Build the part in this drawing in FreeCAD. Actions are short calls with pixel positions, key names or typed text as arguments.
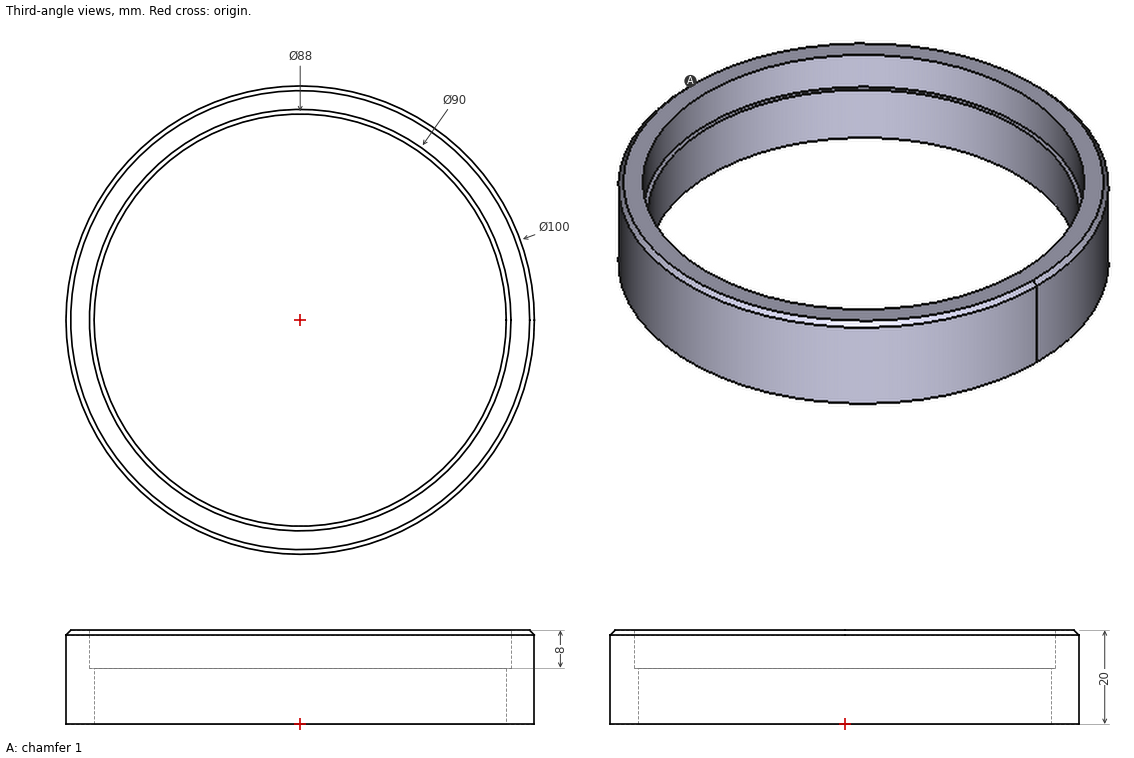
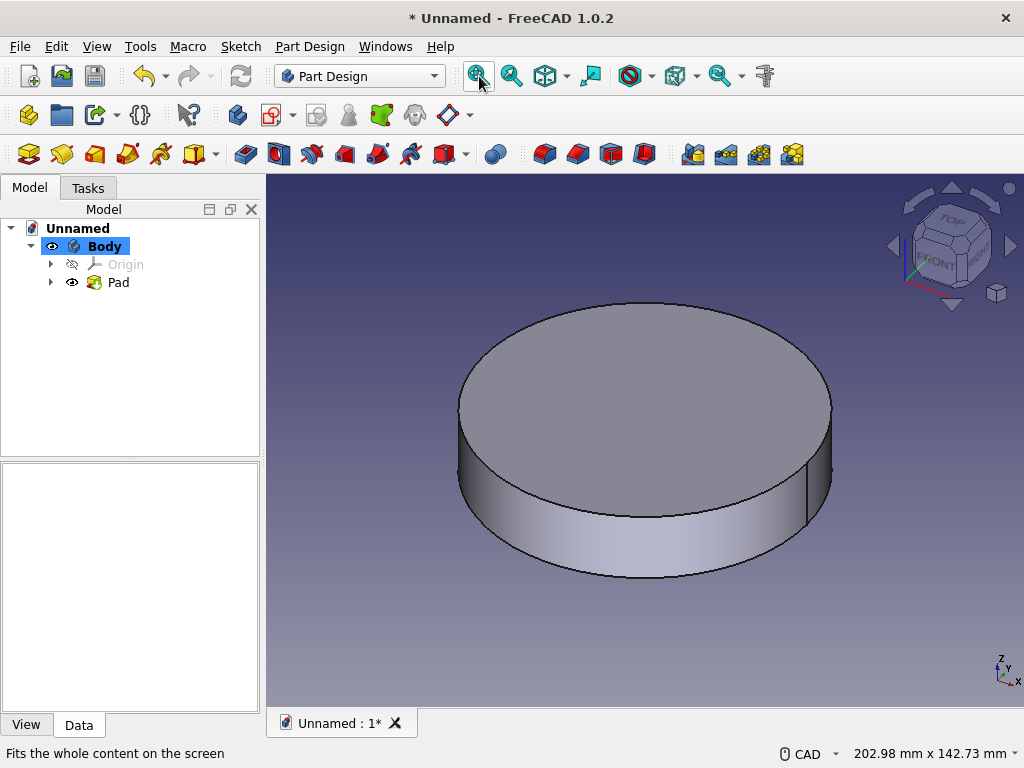
click(645, 409)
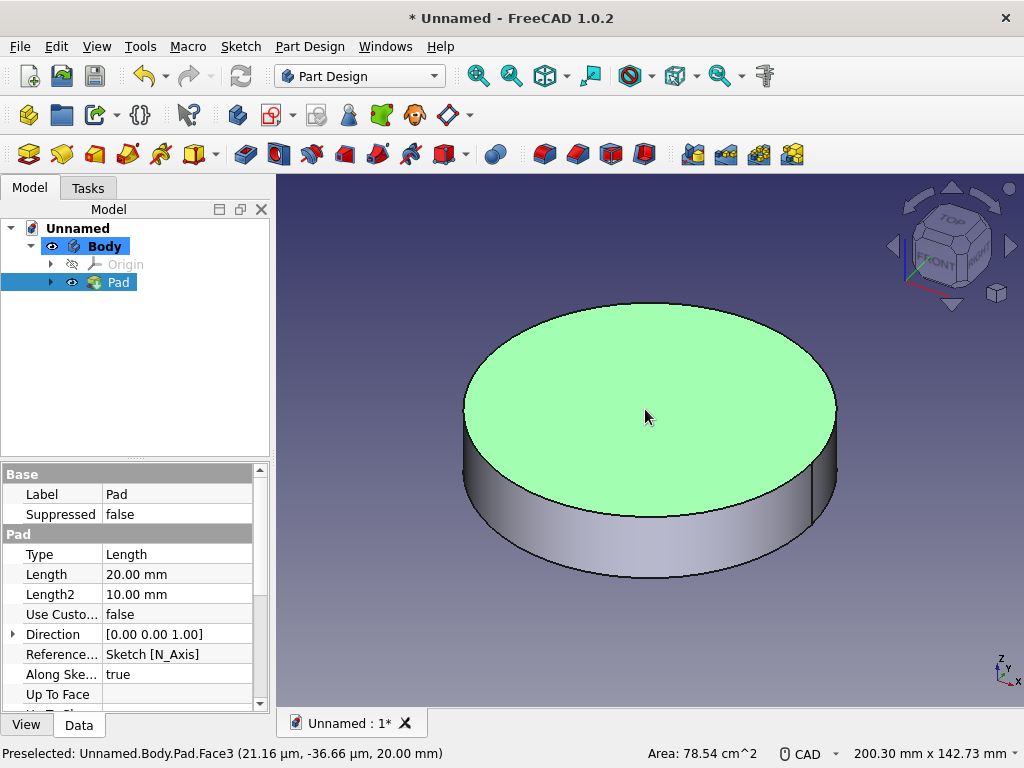
click(270, 116)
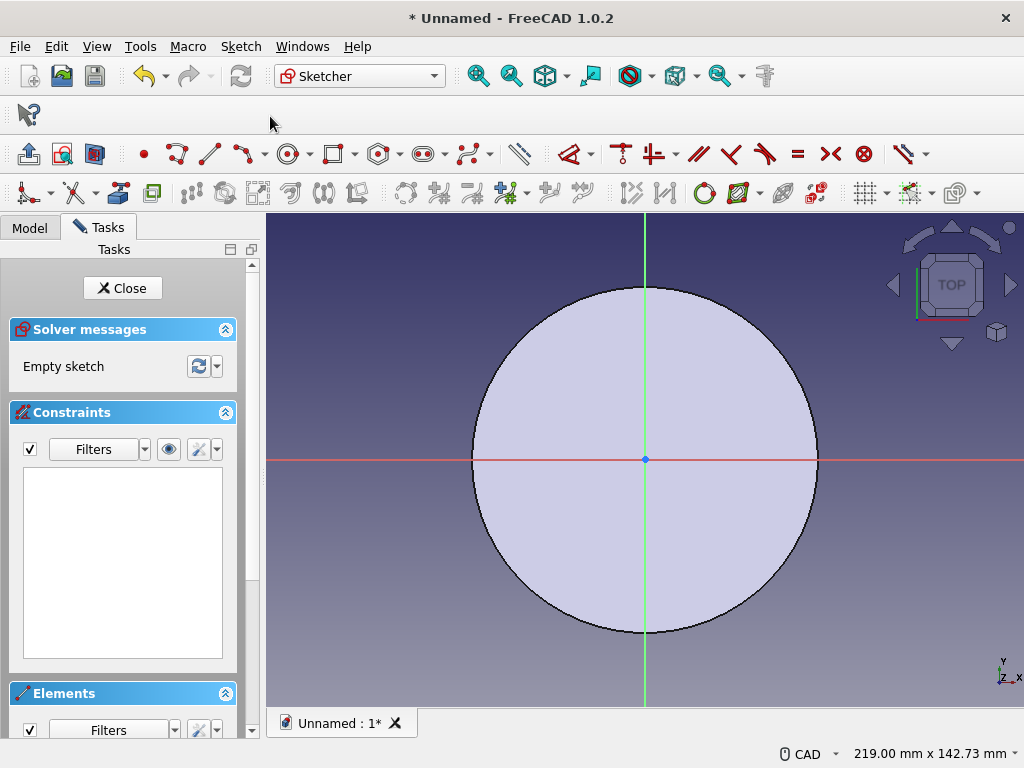
click(288, 154)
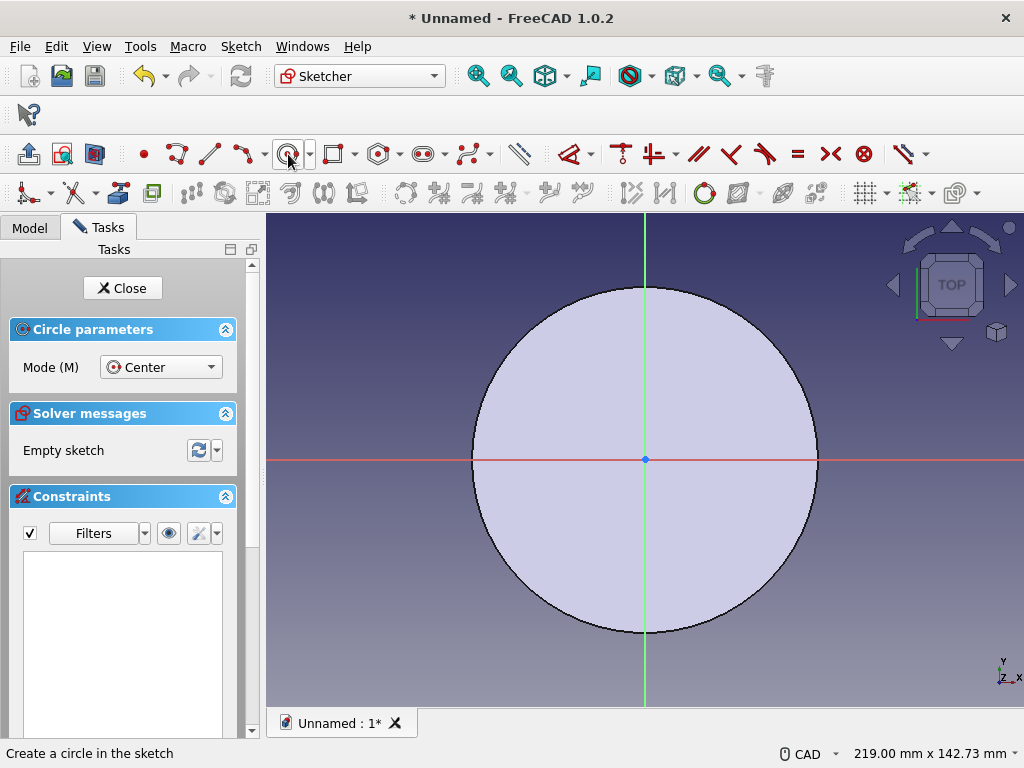
click(645, 460)
move(755, 350)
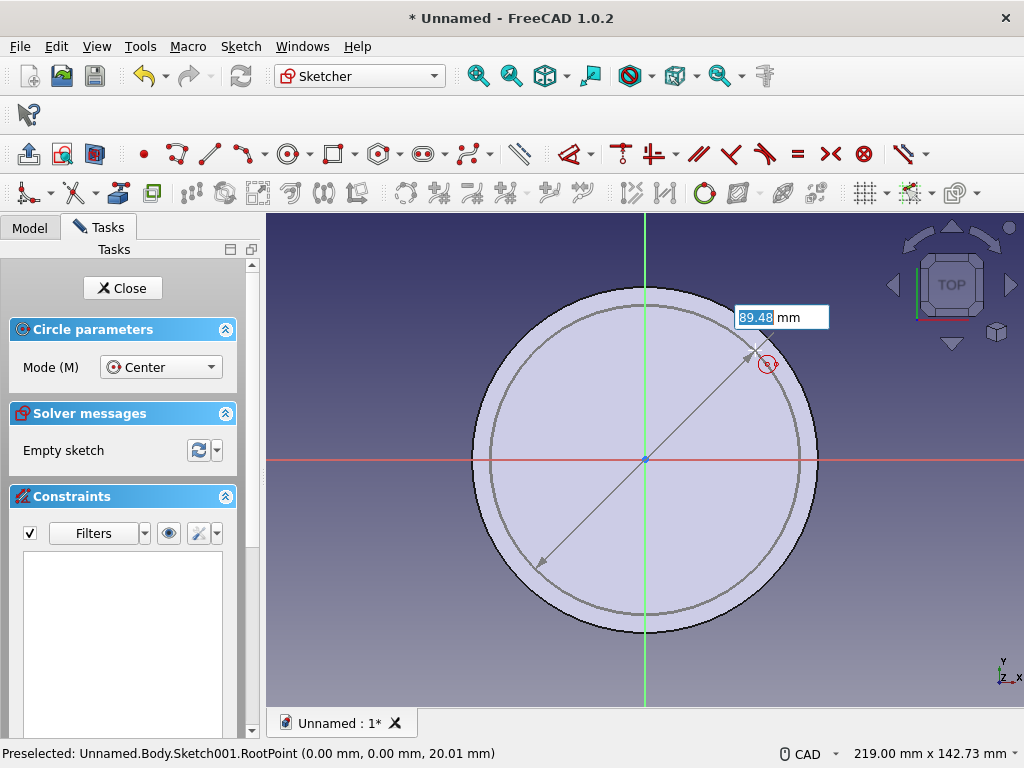
text(90)
key(Return)
key(Escape)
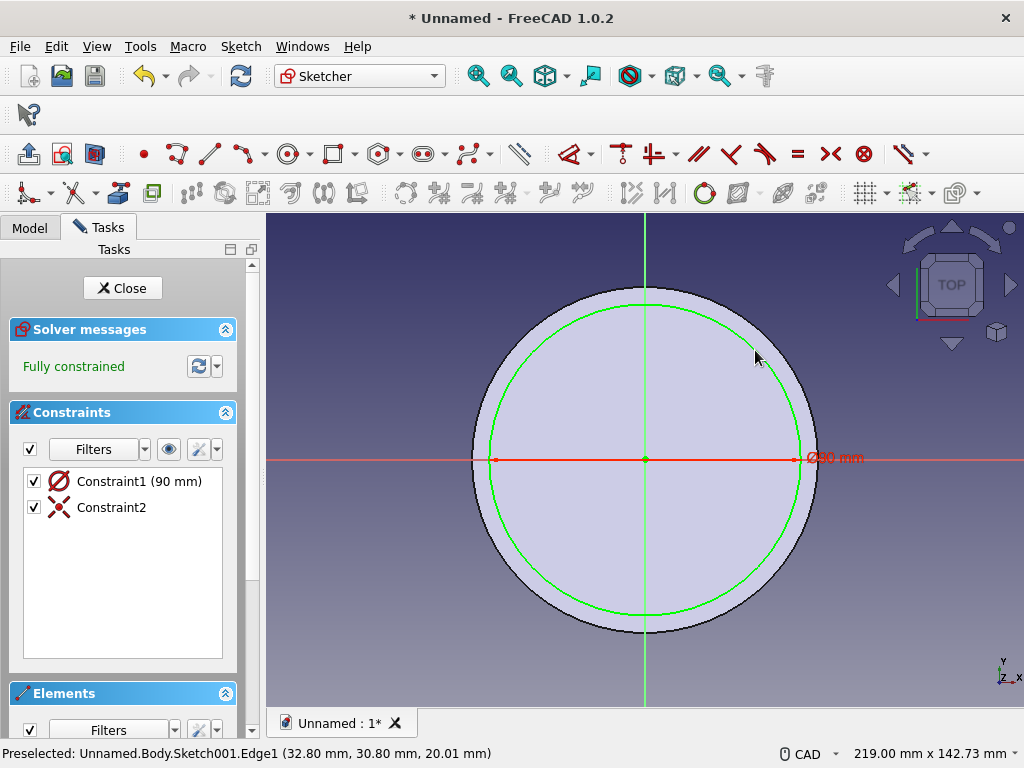
click(123, 288)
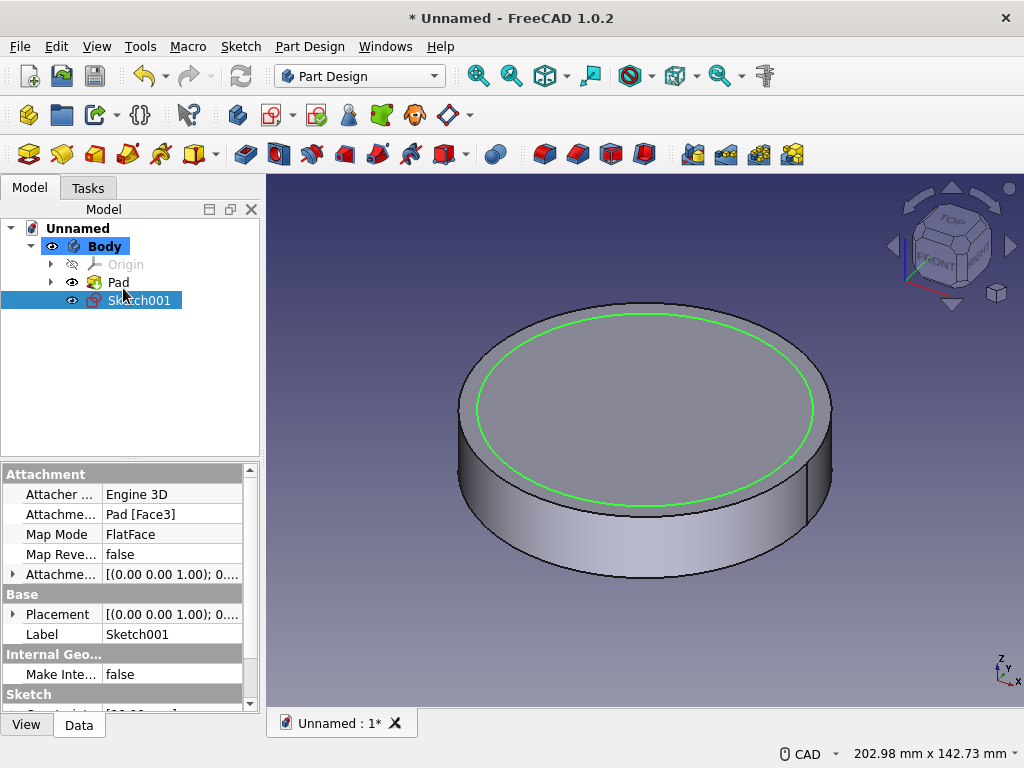
click(246, 154)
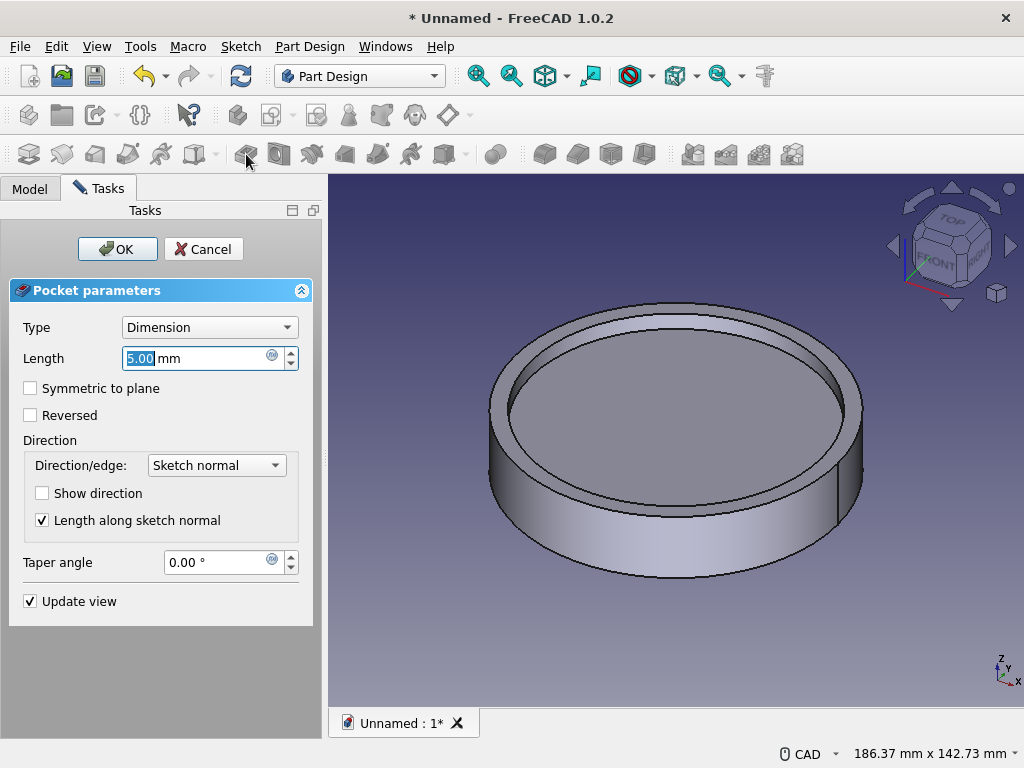
text(8)
key(Tab)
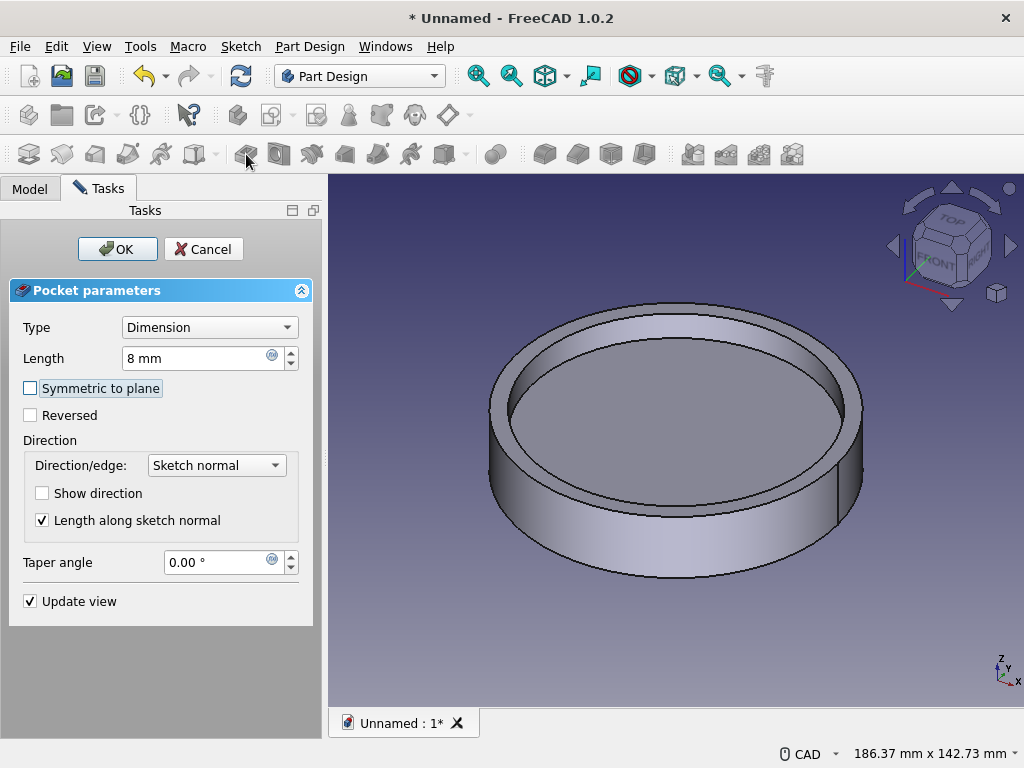
click(118, 249)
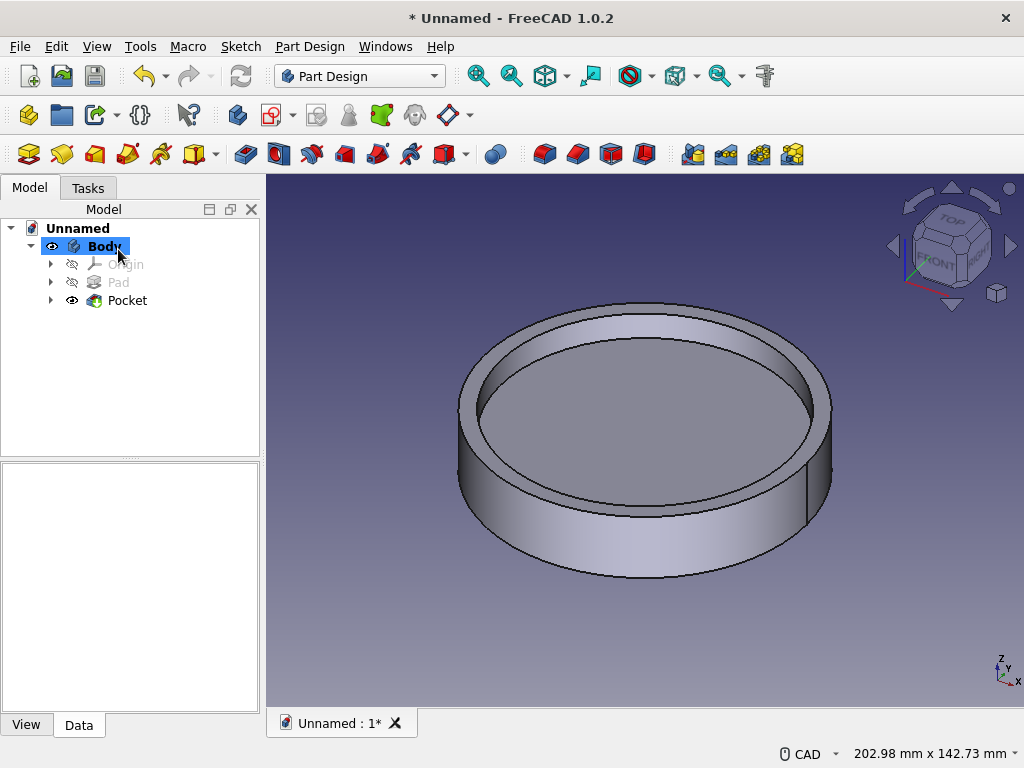
click(645, 433)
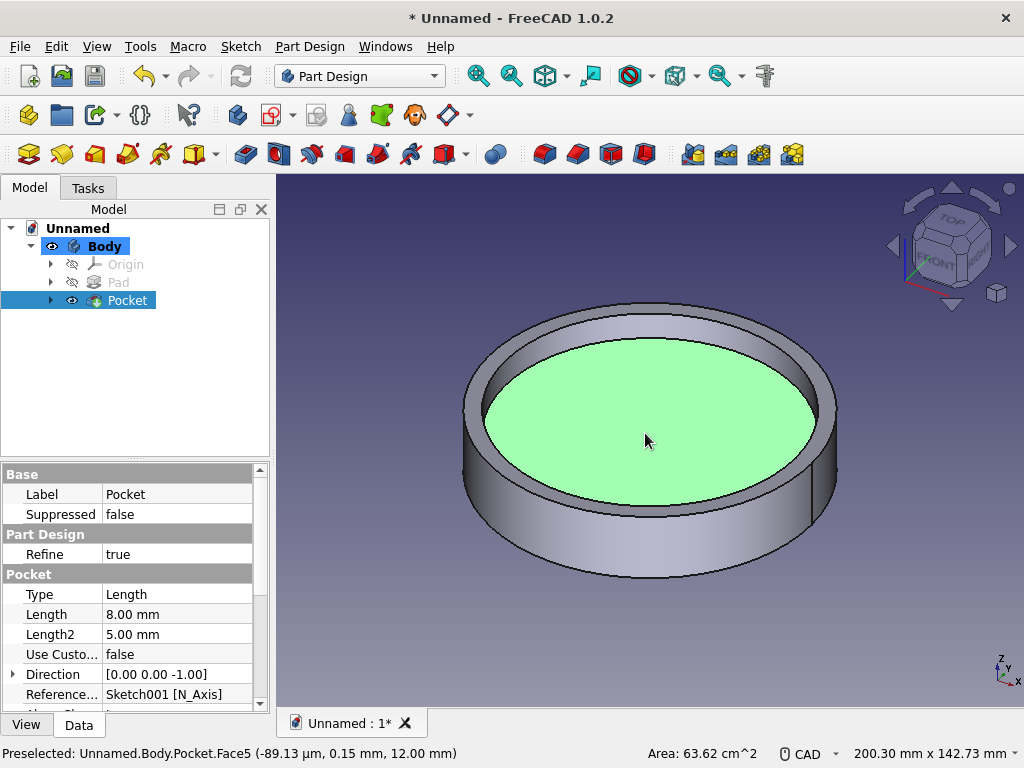
click(270, 116)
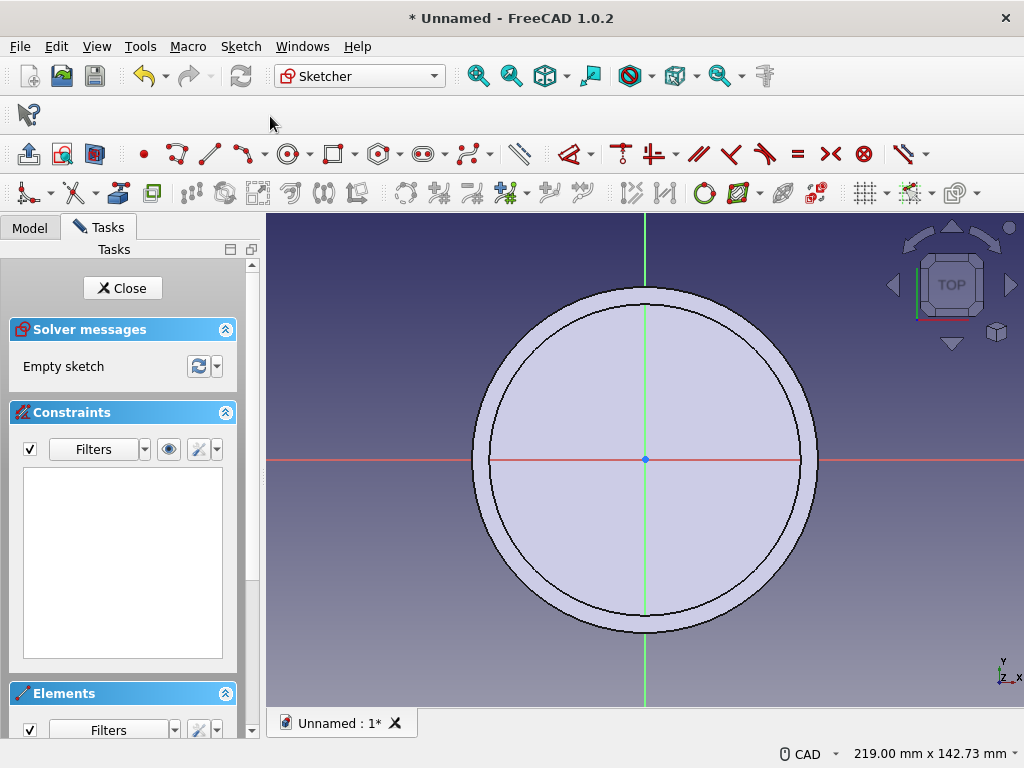
click(288, 154)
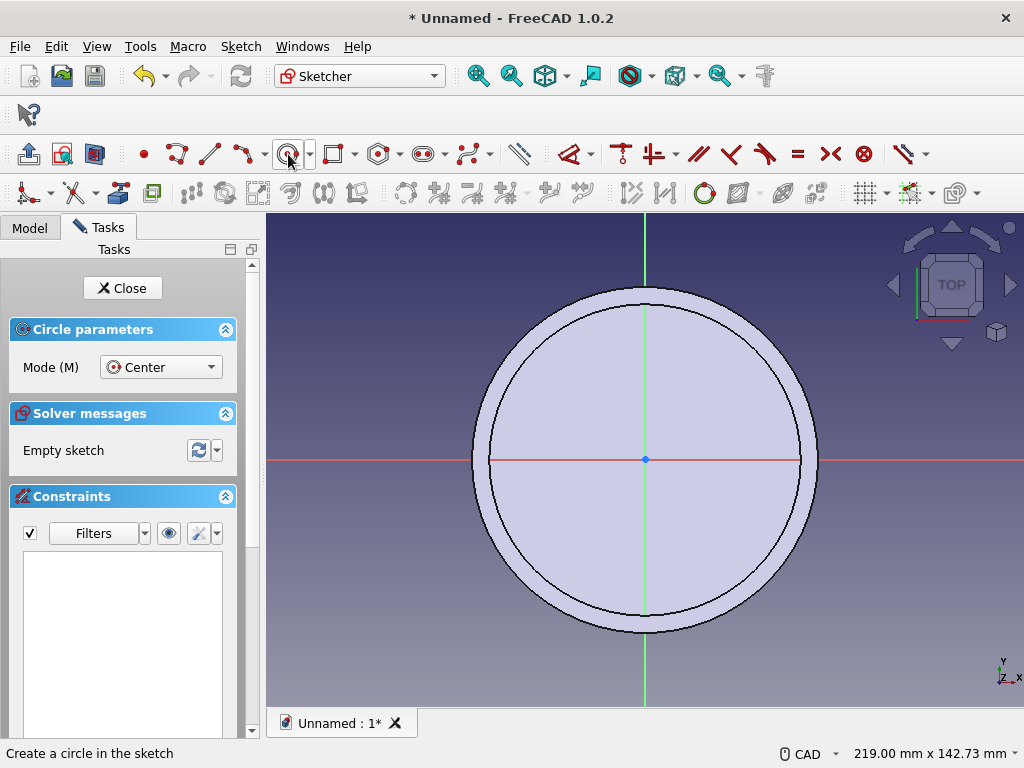
click(645, 460)
move(753, 352)